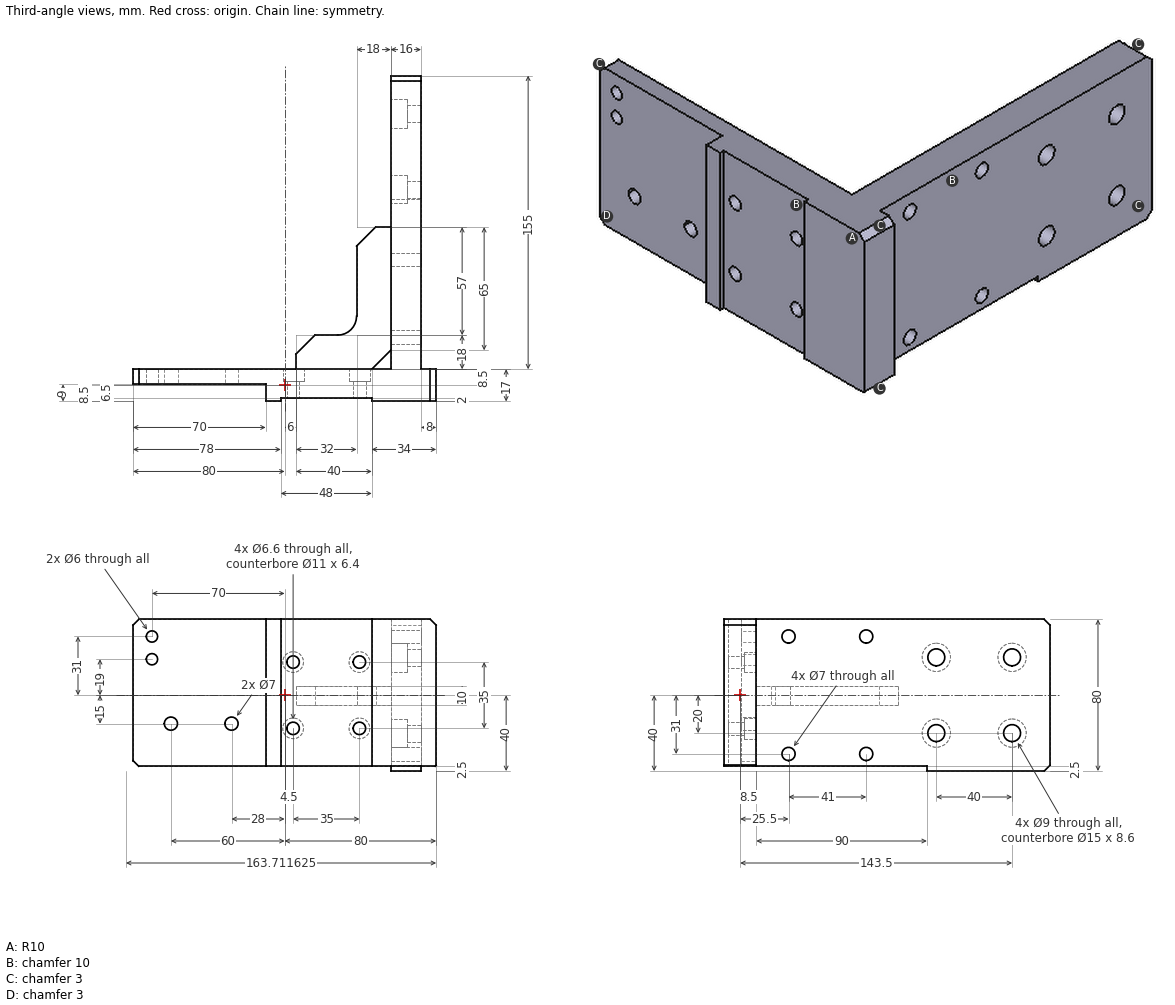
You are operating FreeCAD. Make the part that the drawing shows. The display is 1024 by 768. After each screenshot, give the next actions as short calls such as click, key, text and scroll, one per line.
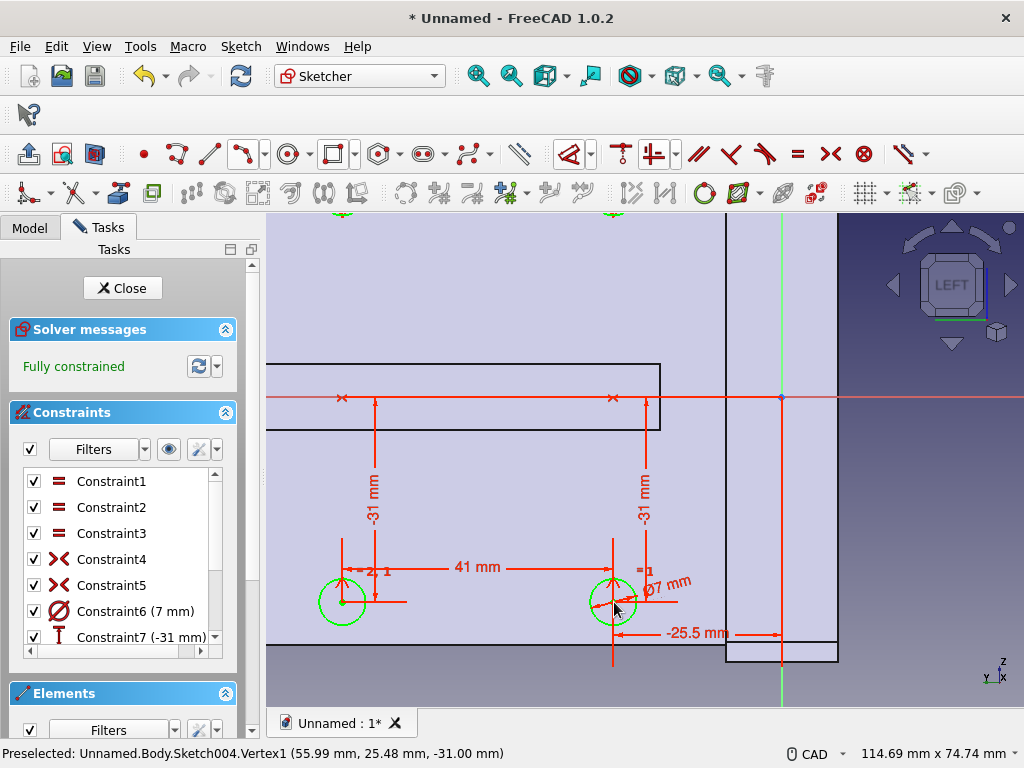
click(123, 288)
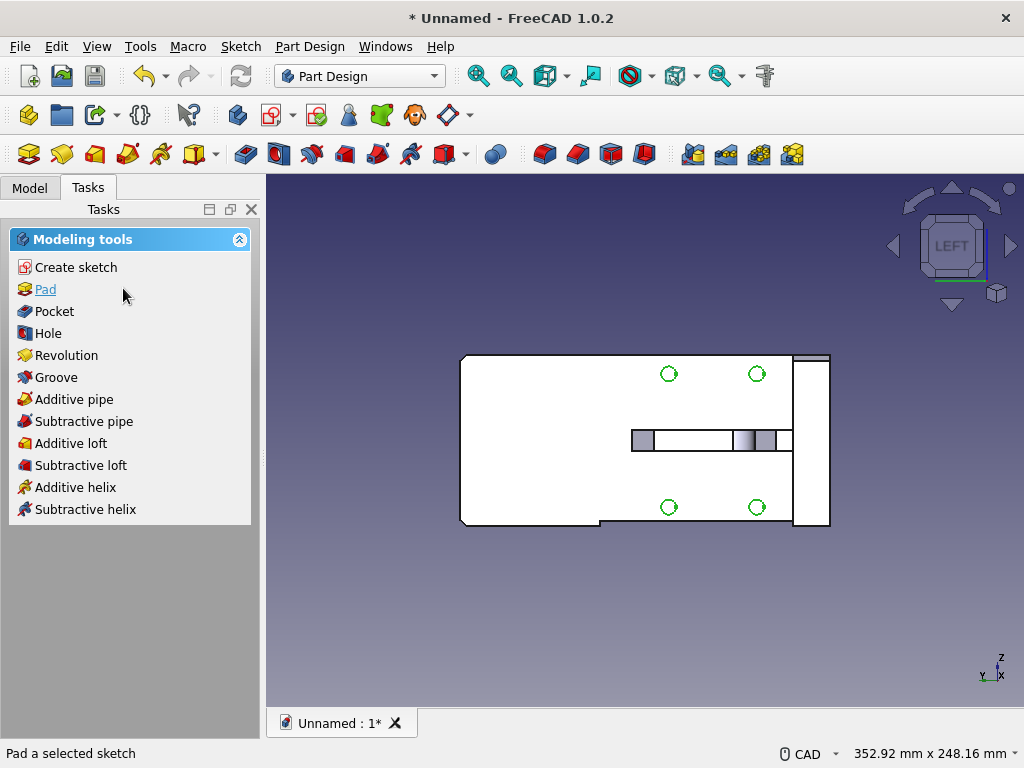
click(279, 154)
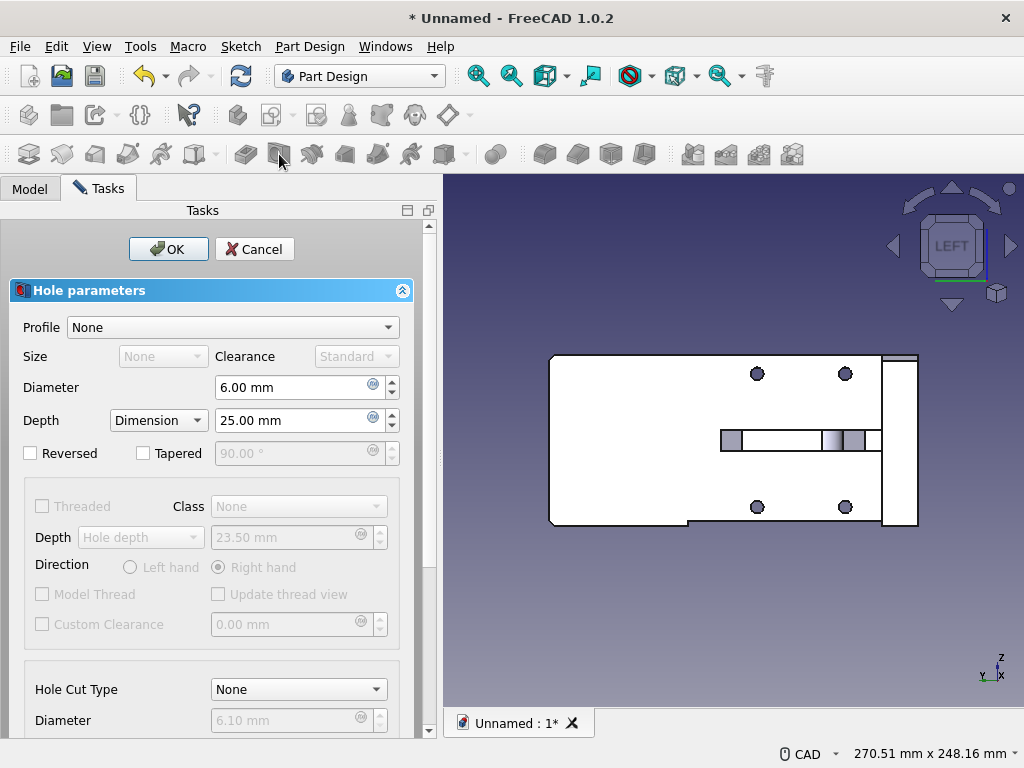
triple_click(300, 388)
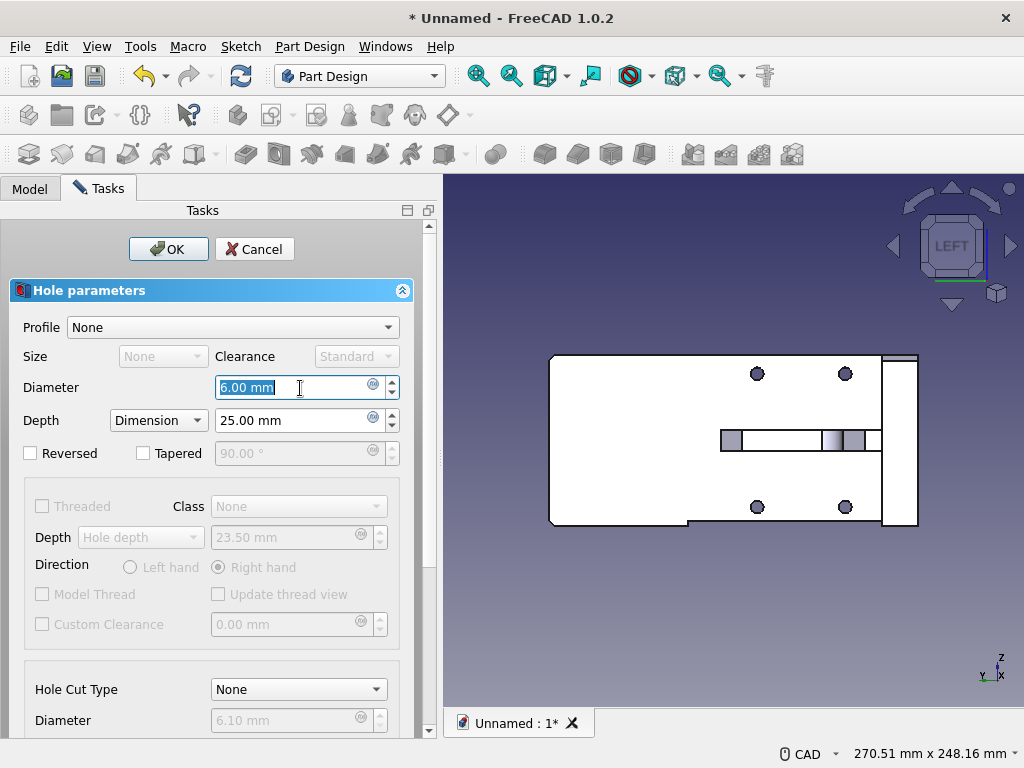
text(7)
key(Tab)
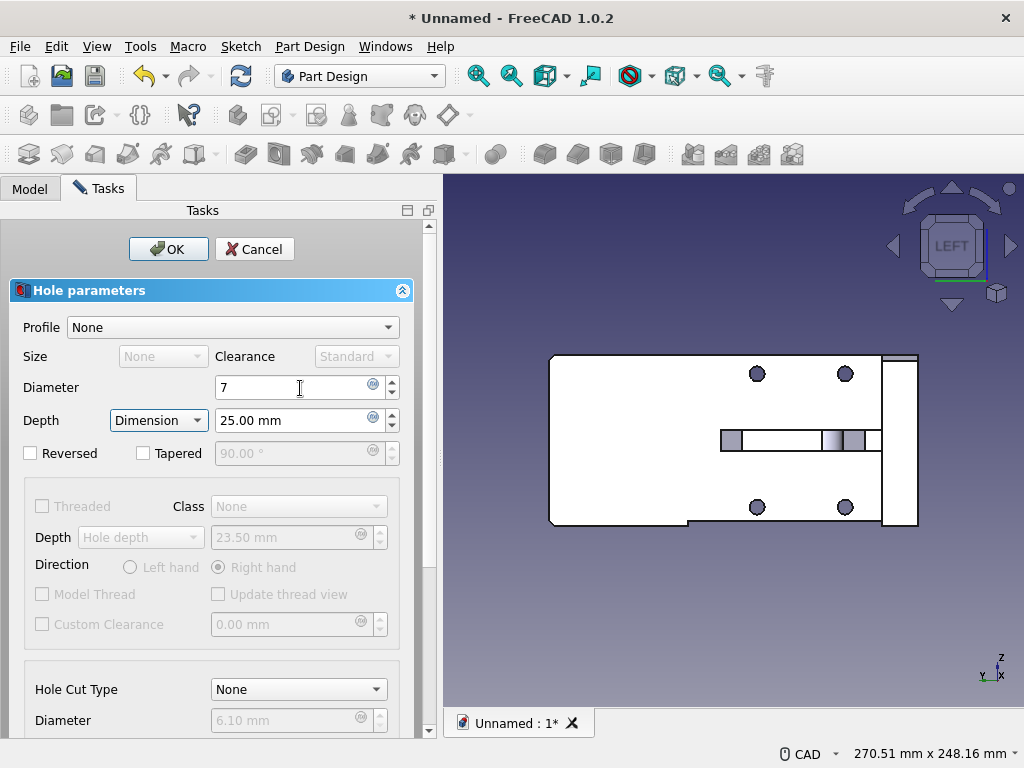
click(160, 420)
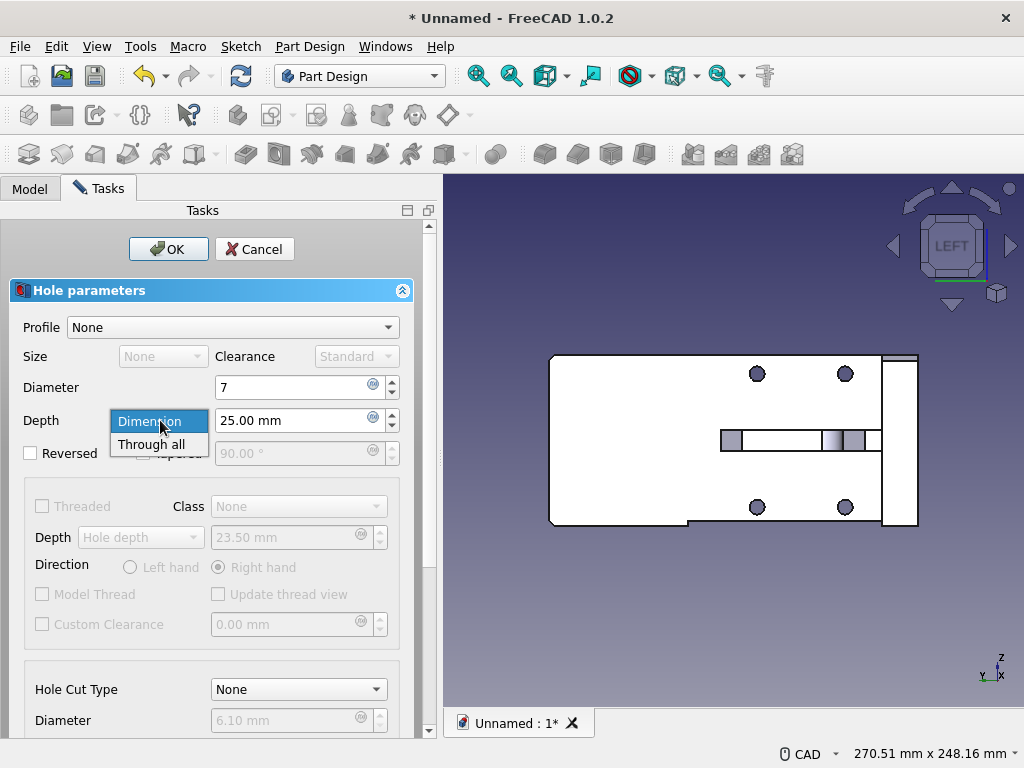
click(158, 444)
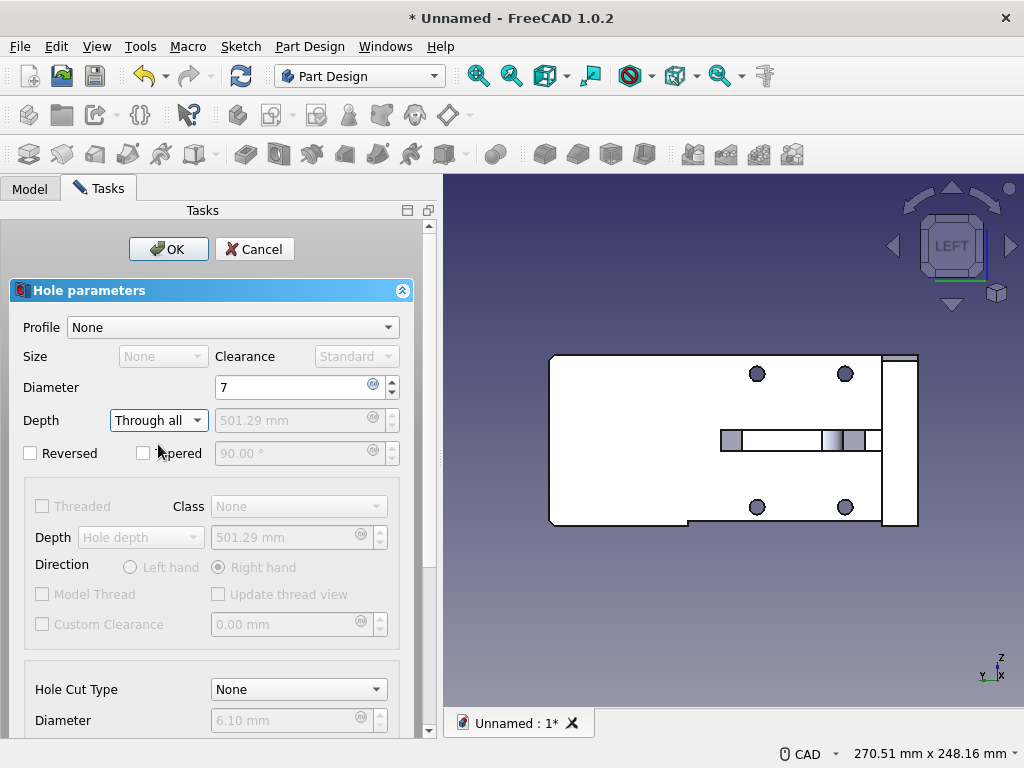
click(169, 249)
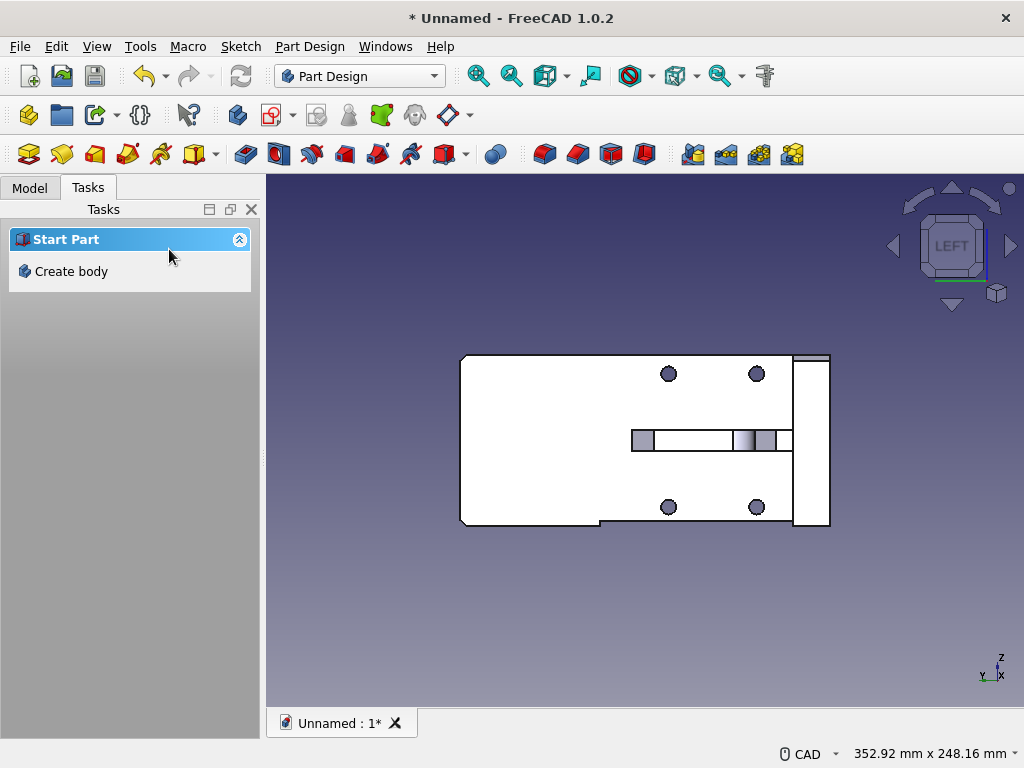
click(532, 440)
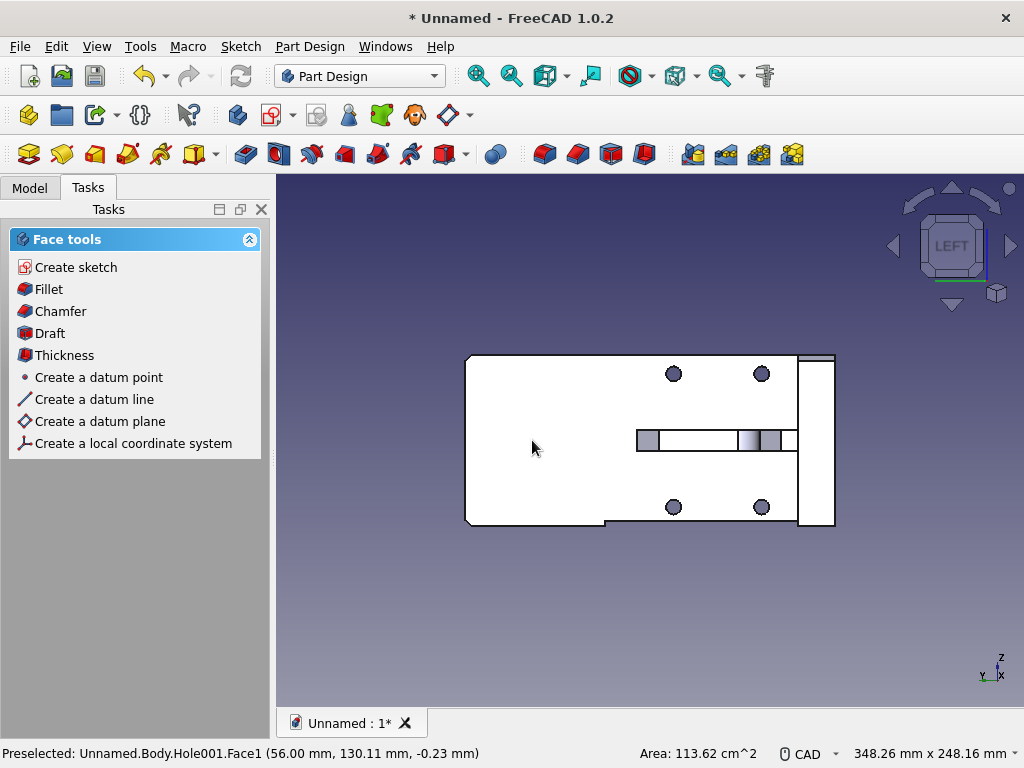
click(270, 116)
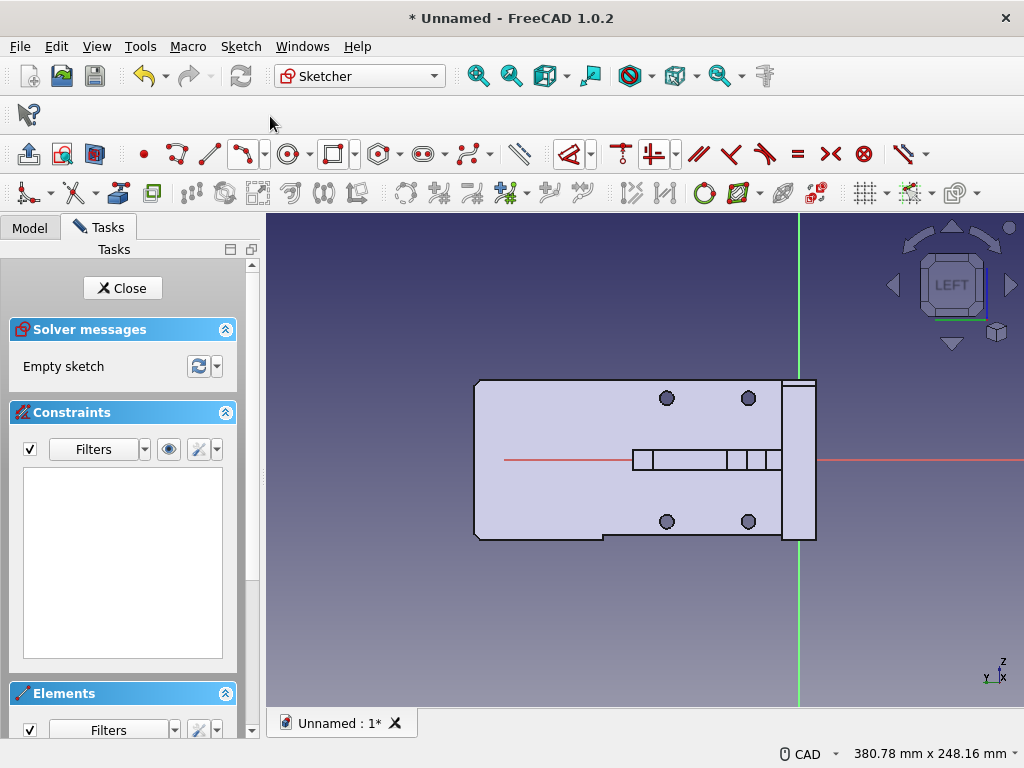
scroll(543, 460, up, 6)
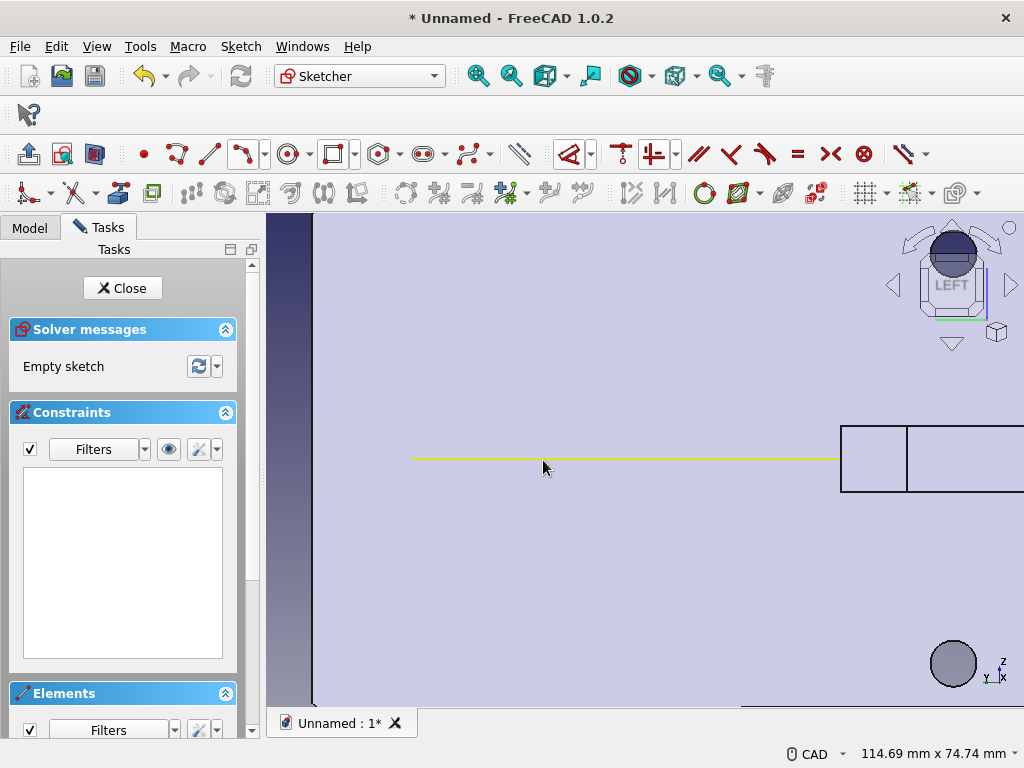
click(288, 154)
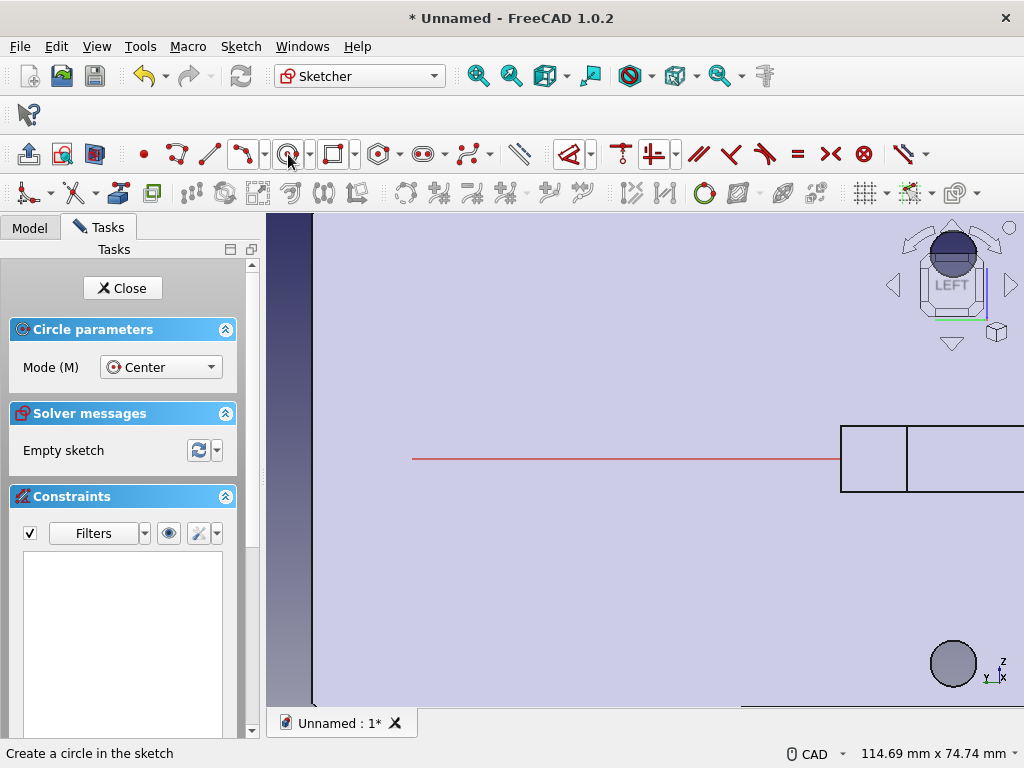
click(445, 591)
click(466, 570)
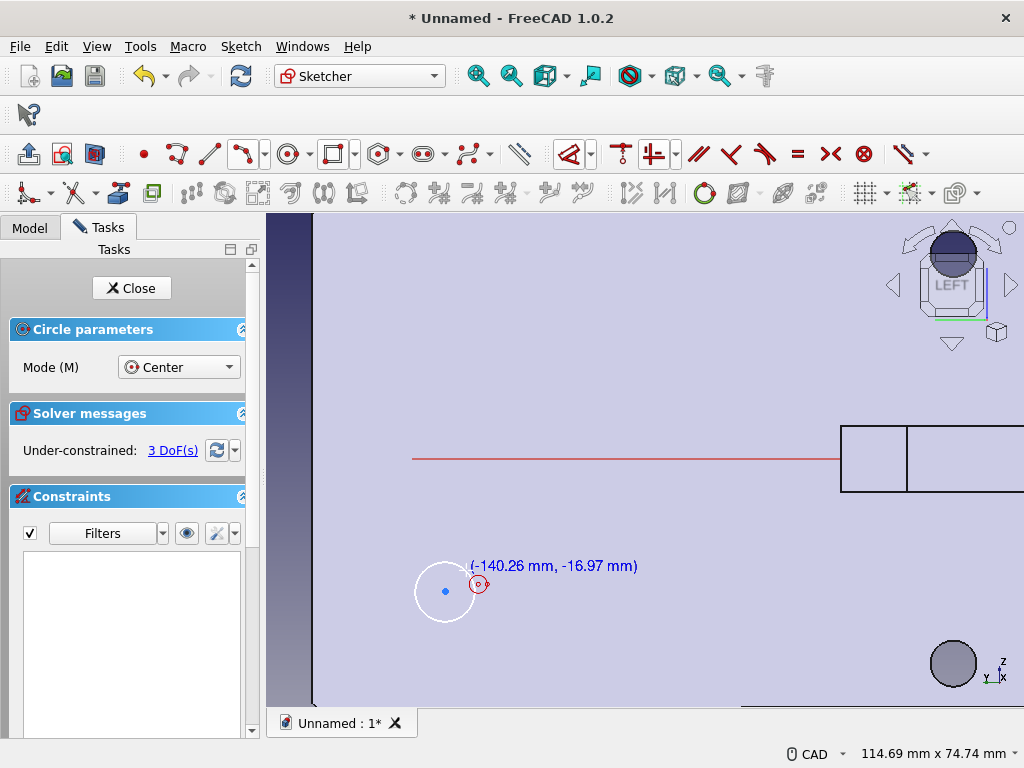
click(709, 591)
click(730, 570)